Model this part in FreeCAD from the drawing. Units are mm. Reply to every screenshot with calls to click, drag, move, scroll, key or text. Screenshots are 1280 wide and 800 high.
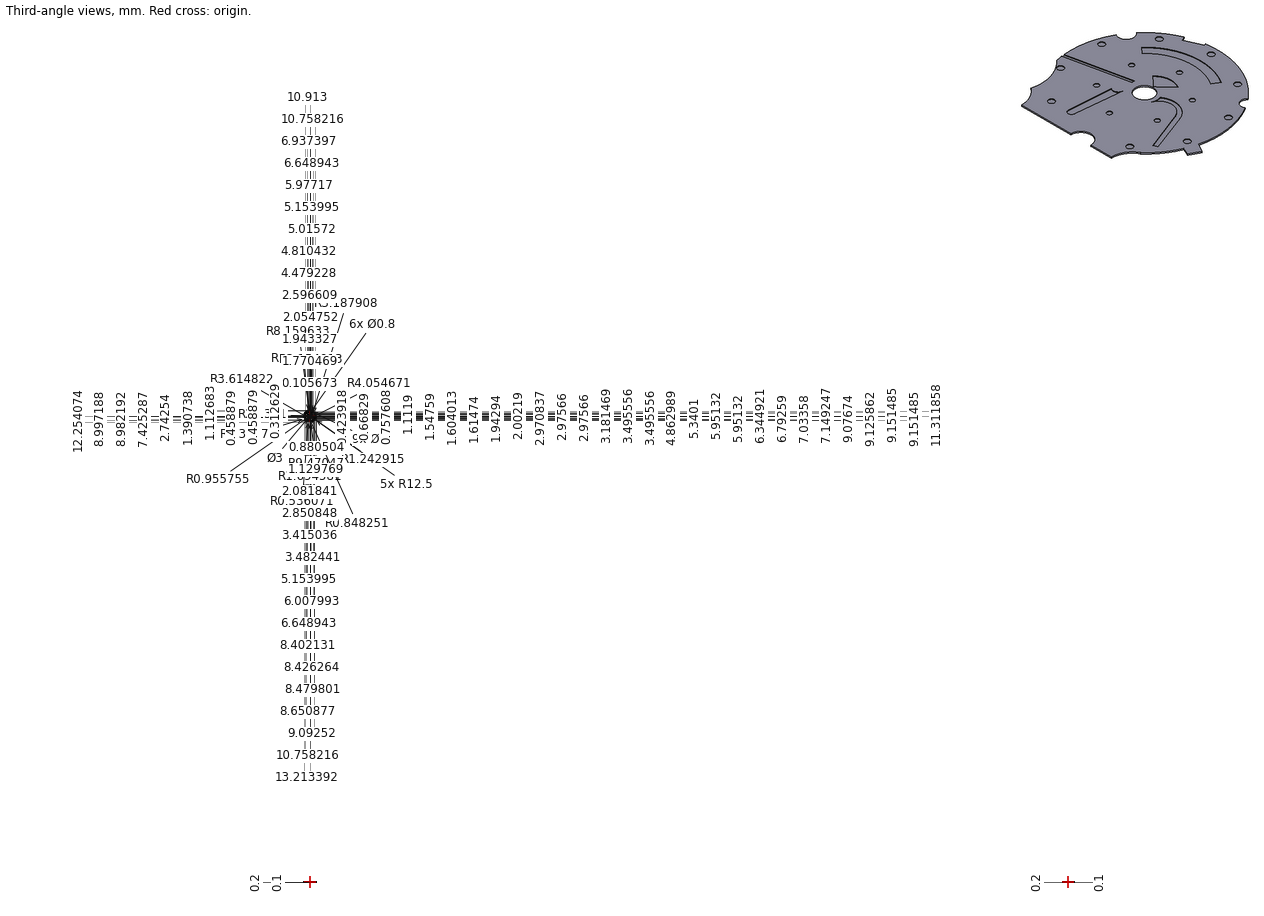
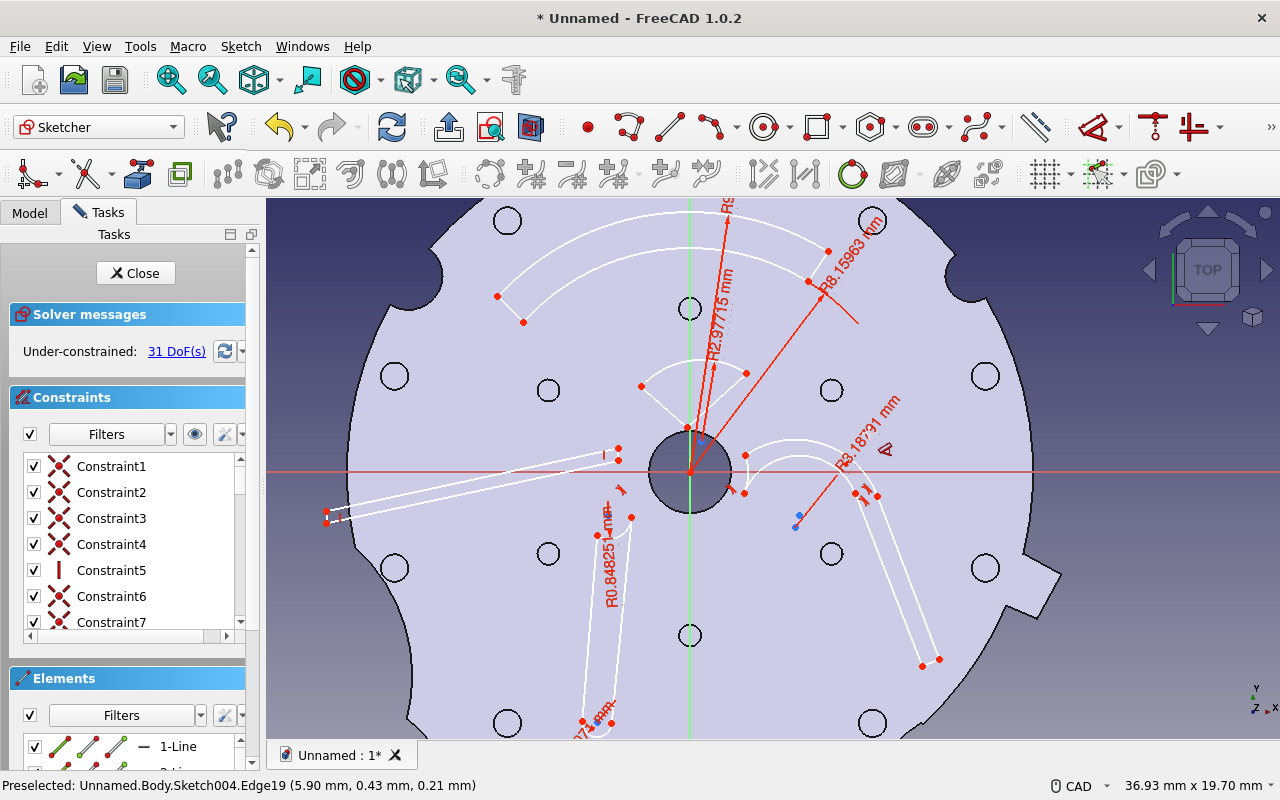
scroll(747, 463, up, 3)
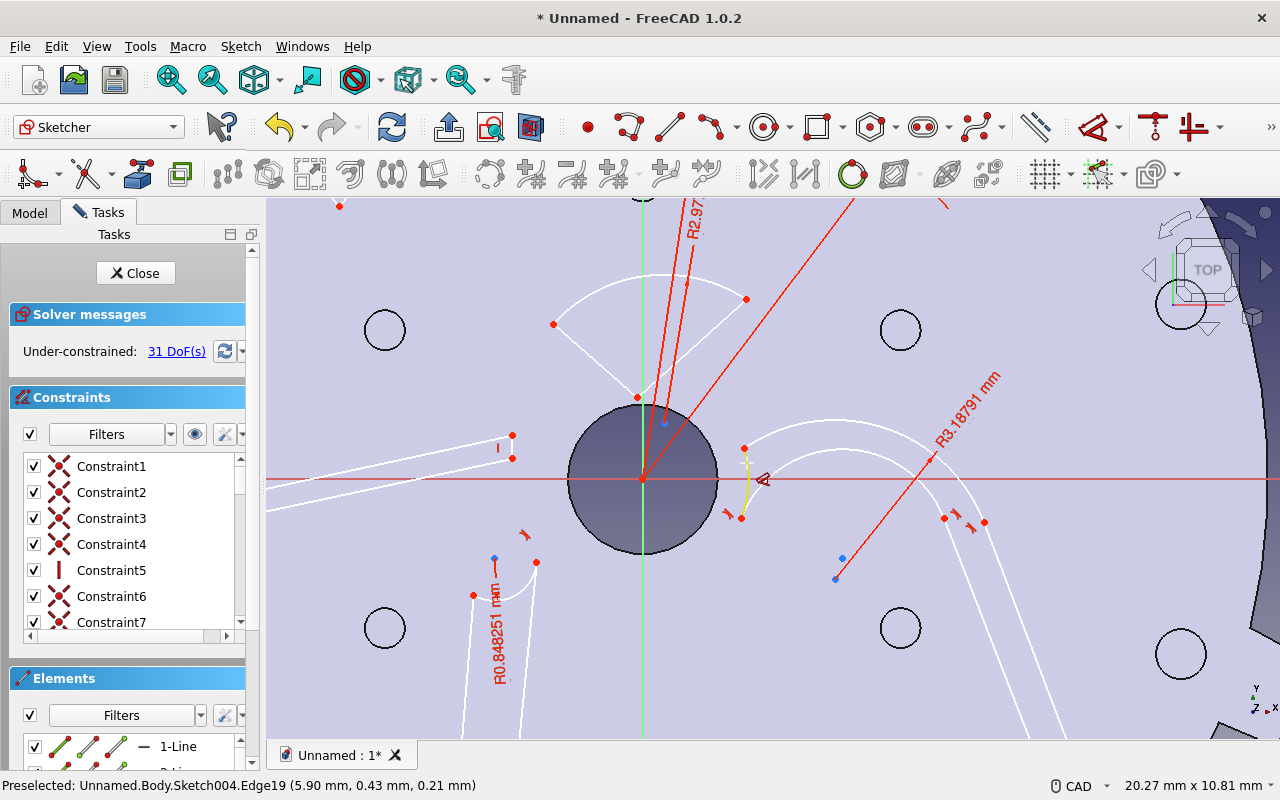
click(747, 462)
click(773, 525)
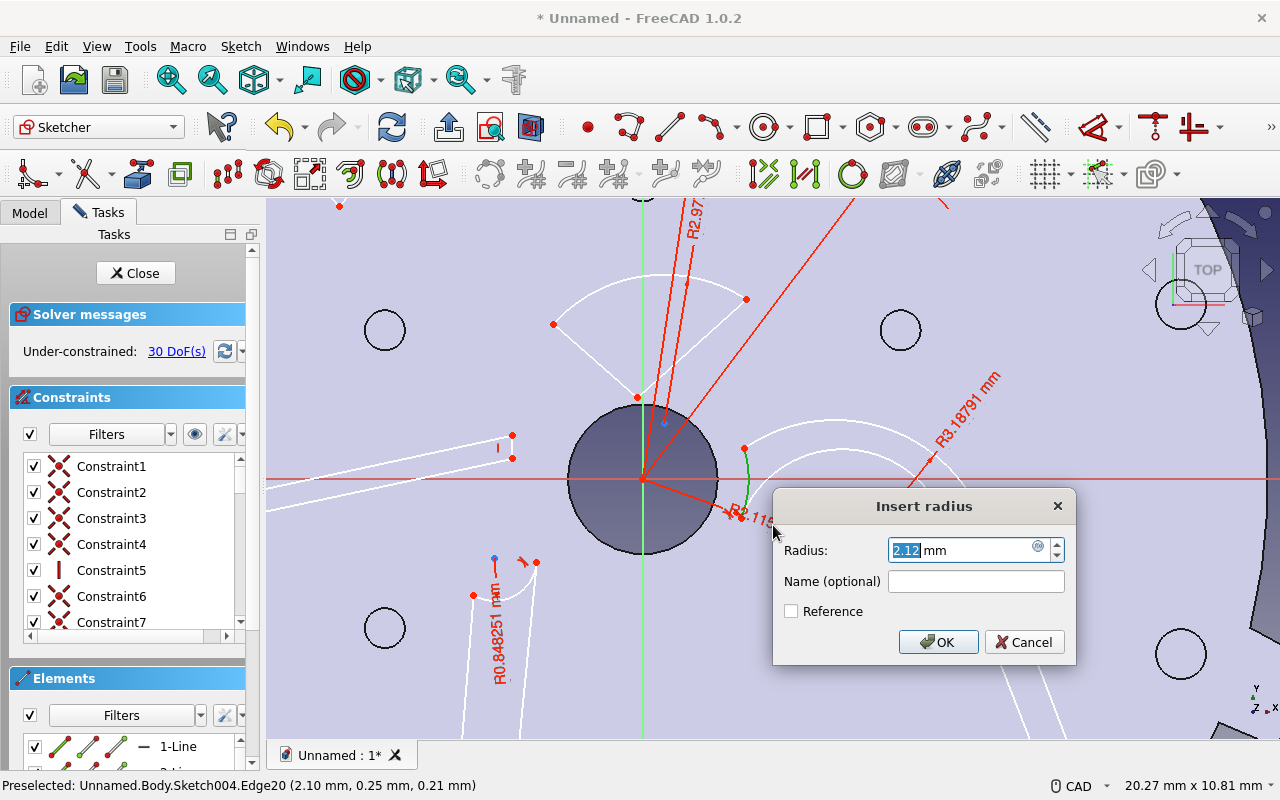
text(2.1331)
key(Return)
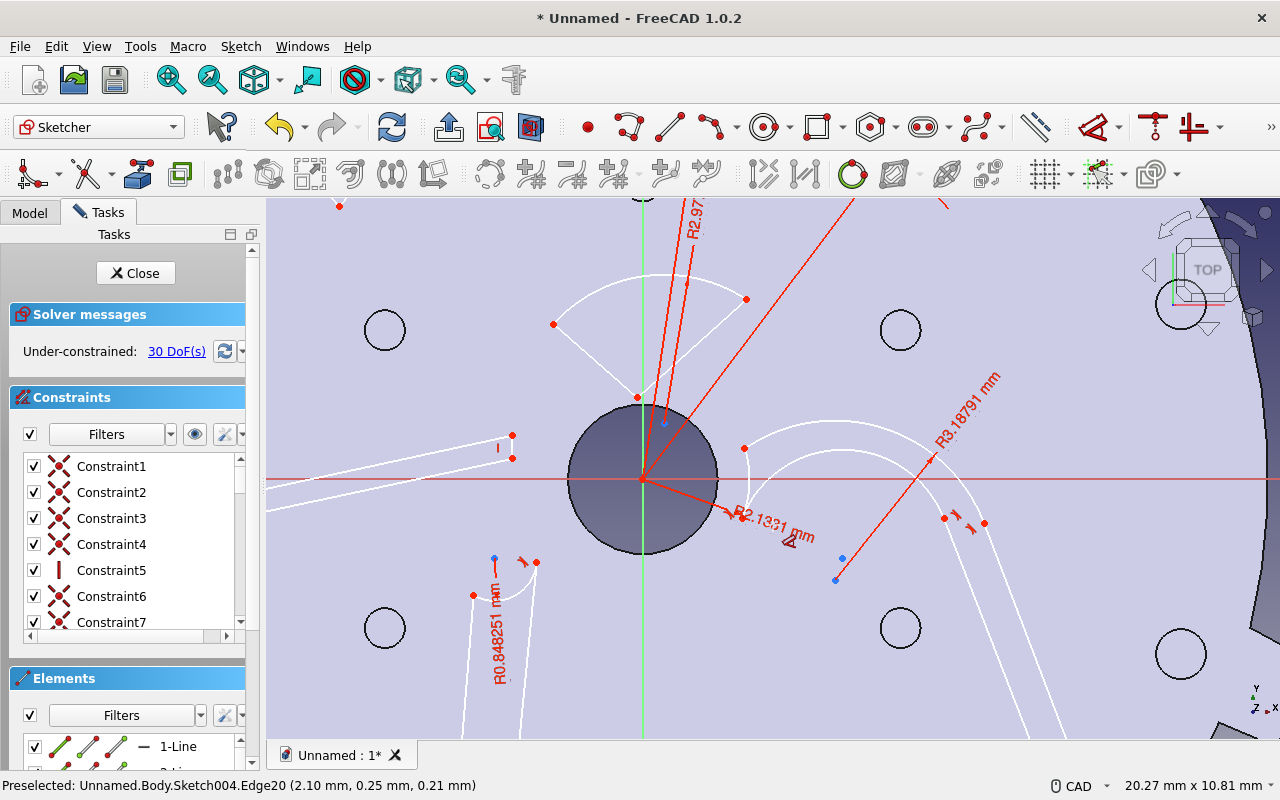
click(893, 462)
click(968, 623)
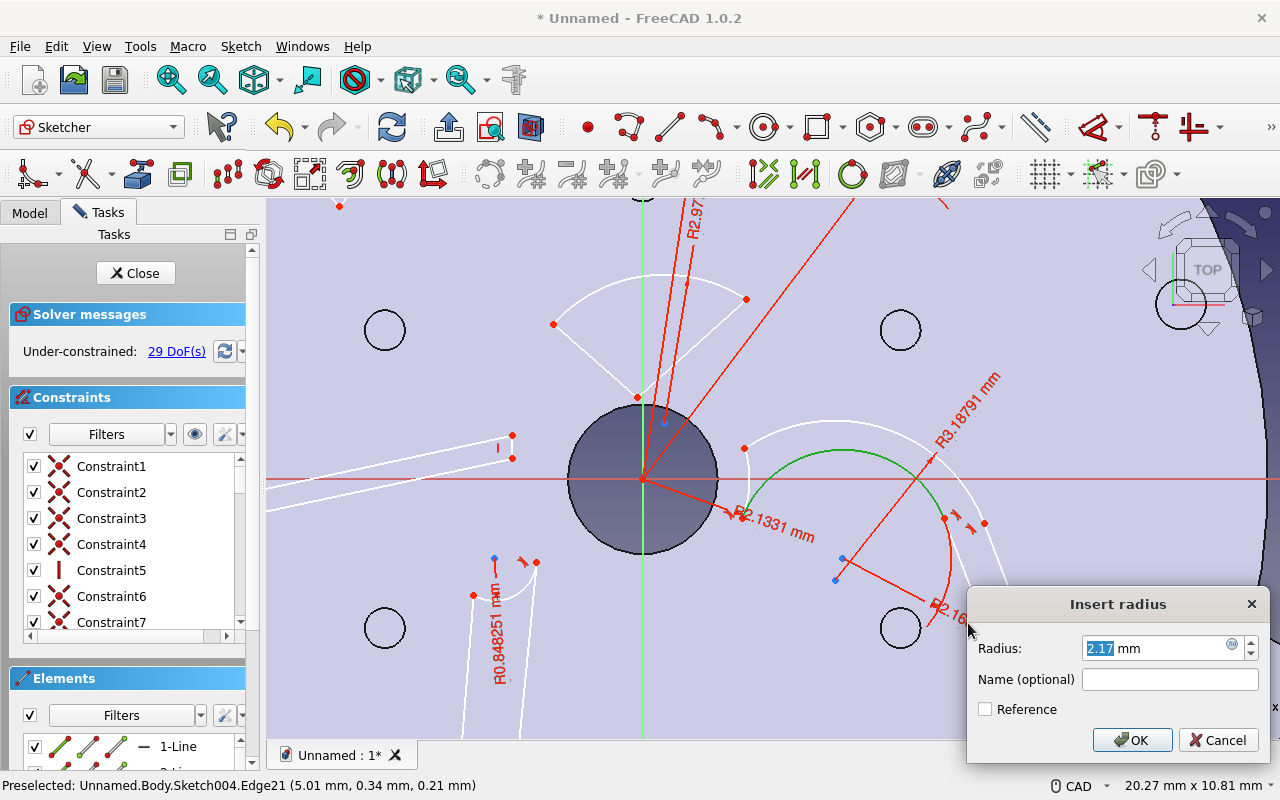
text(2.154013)
key(Return)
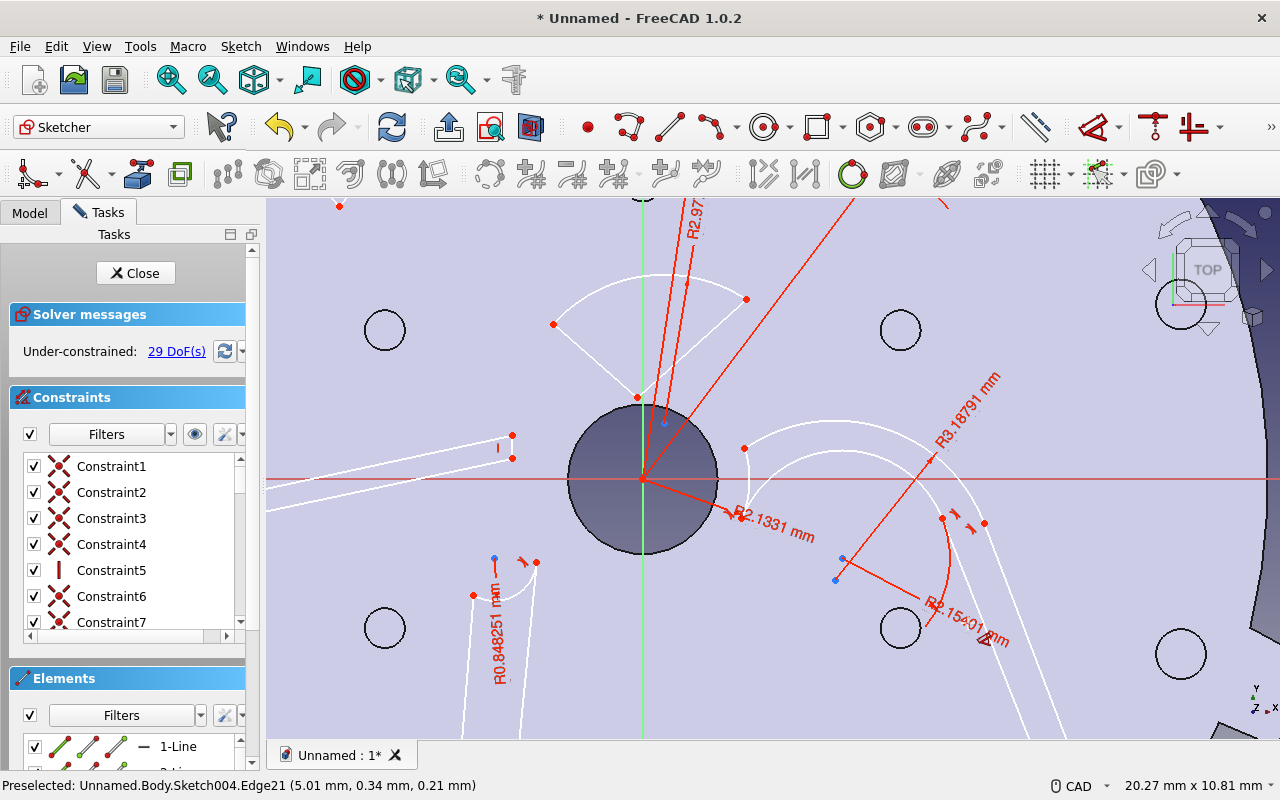
scroll(800, 460, down, 5)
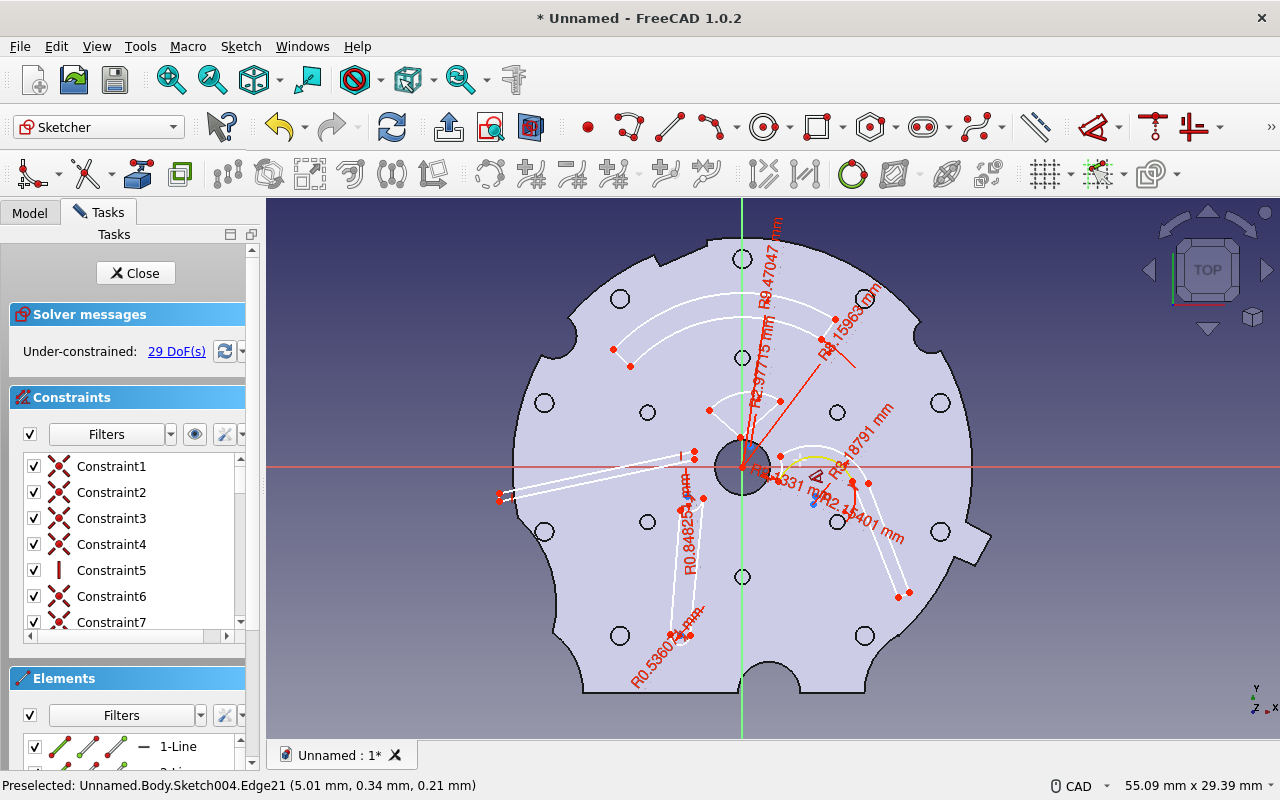
scroll(826, 334, up, 4)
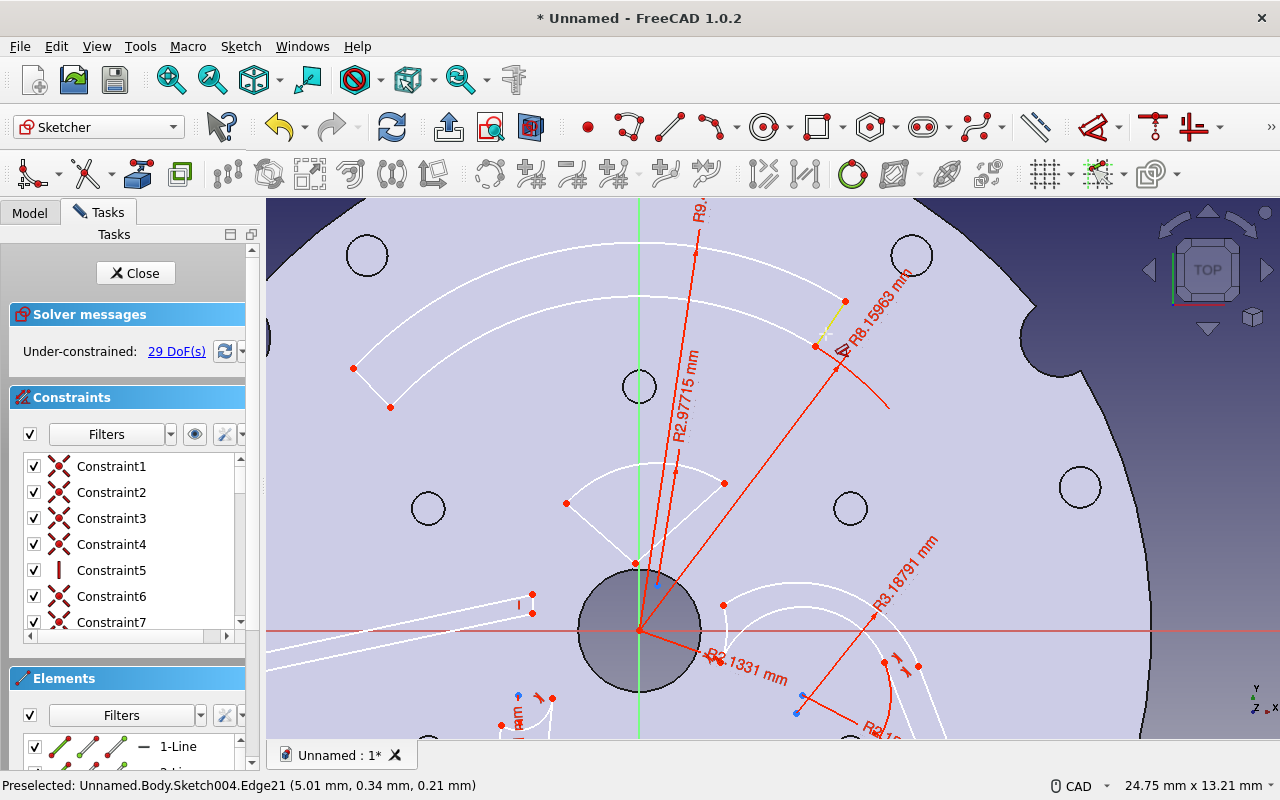
click(825, 333)
click(880, 334)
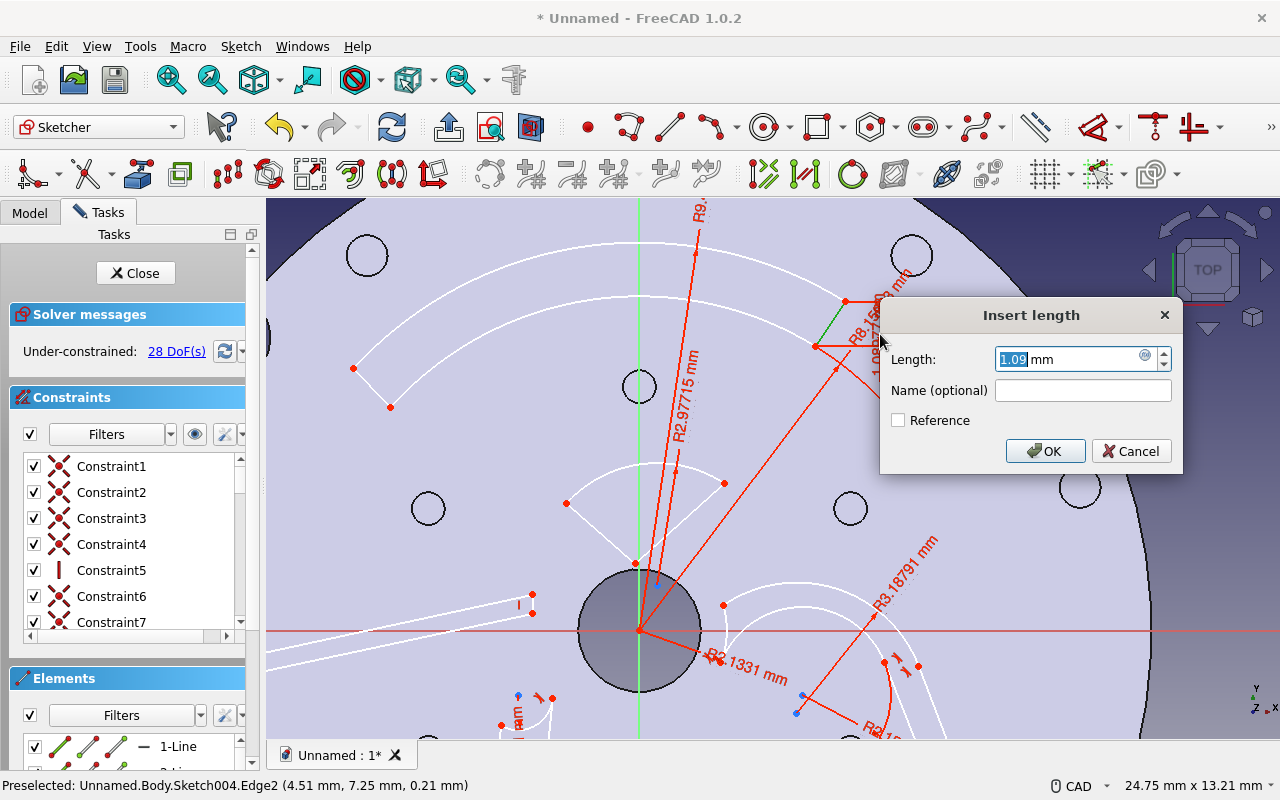
text(1.1119)
key(Return)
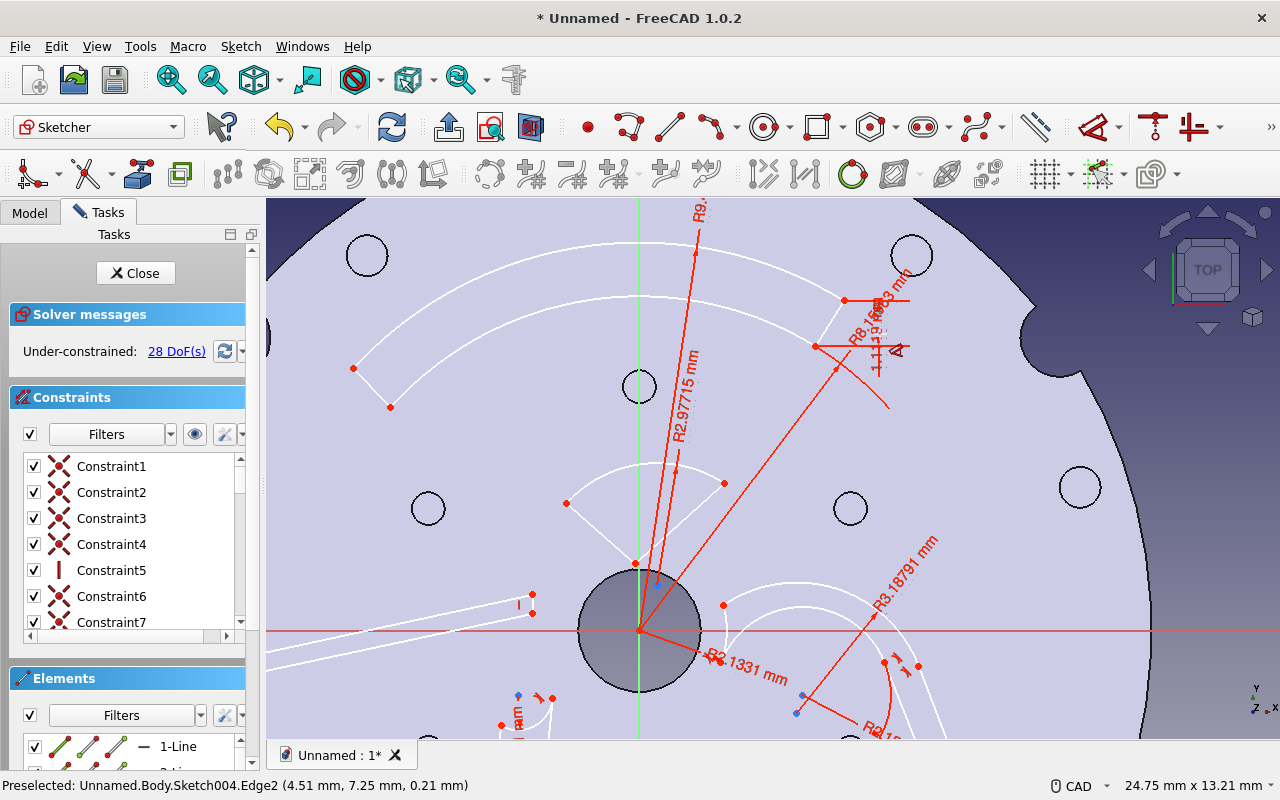
scroll(533, 604, up, 4)